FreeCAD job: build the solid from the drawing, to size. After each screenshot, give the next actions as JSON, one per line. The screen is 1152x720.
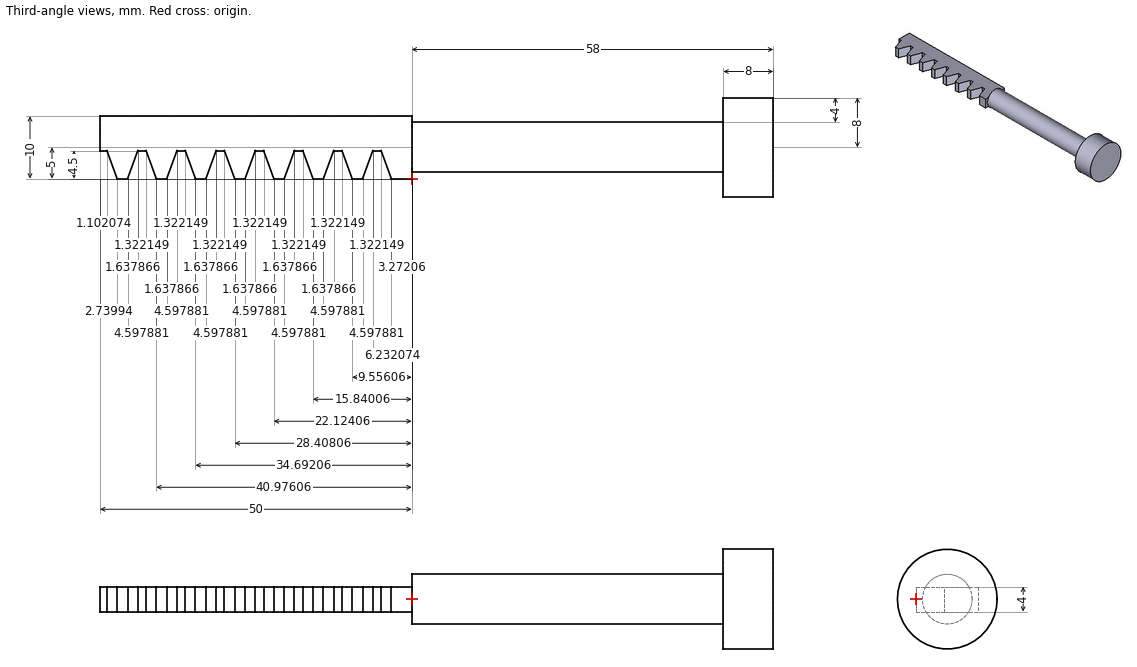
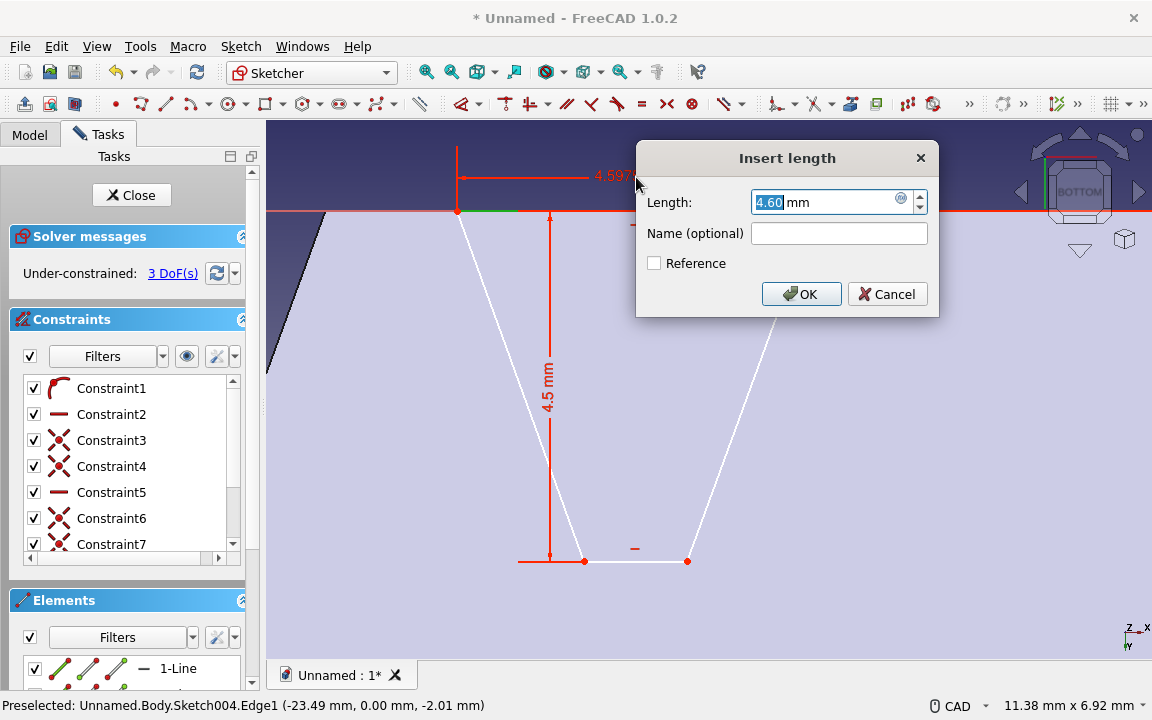
{"action": "type", "text": "4.597881"}
{"action": "key", "text": "Return"}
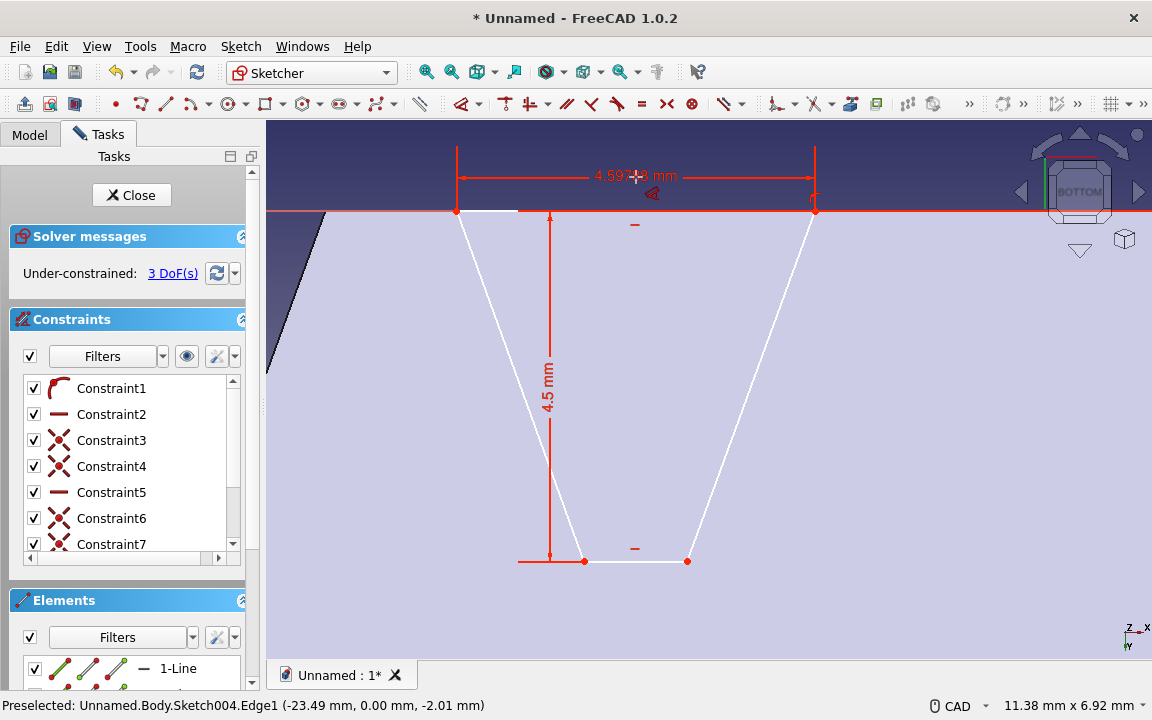
{"action": "left_click", "coordinate": [615, 562]}
{"action": "left_click", "coordinate": [635, 596]}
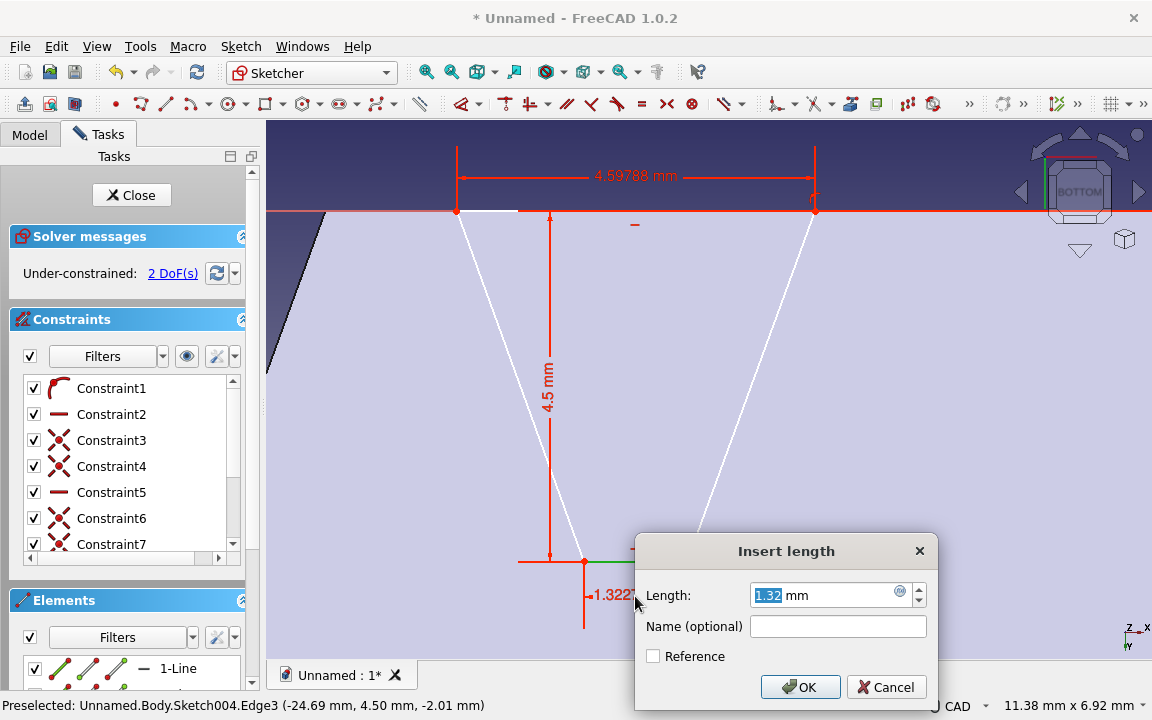
{"action": "type", "text": "1.322149"}
{"action": "key", "text": "Return"}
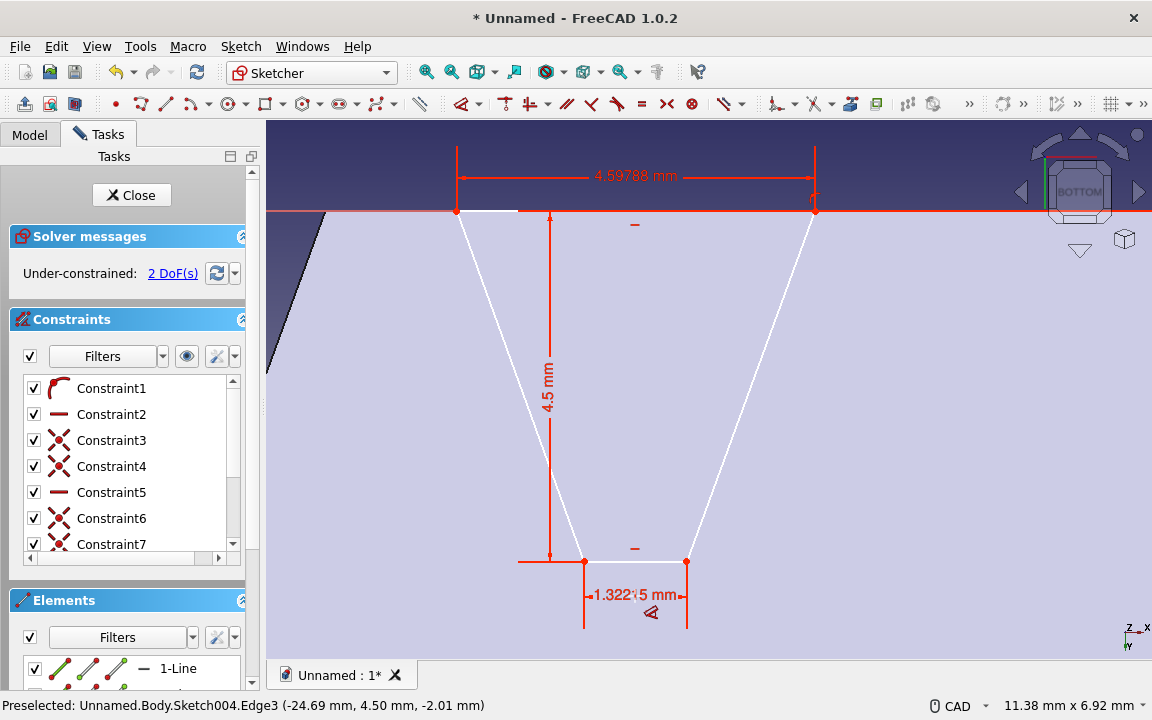
{"action": "left_click", "coordinate": [815, 211]}
{"action": "left_click", "coordinate": [901, 177]}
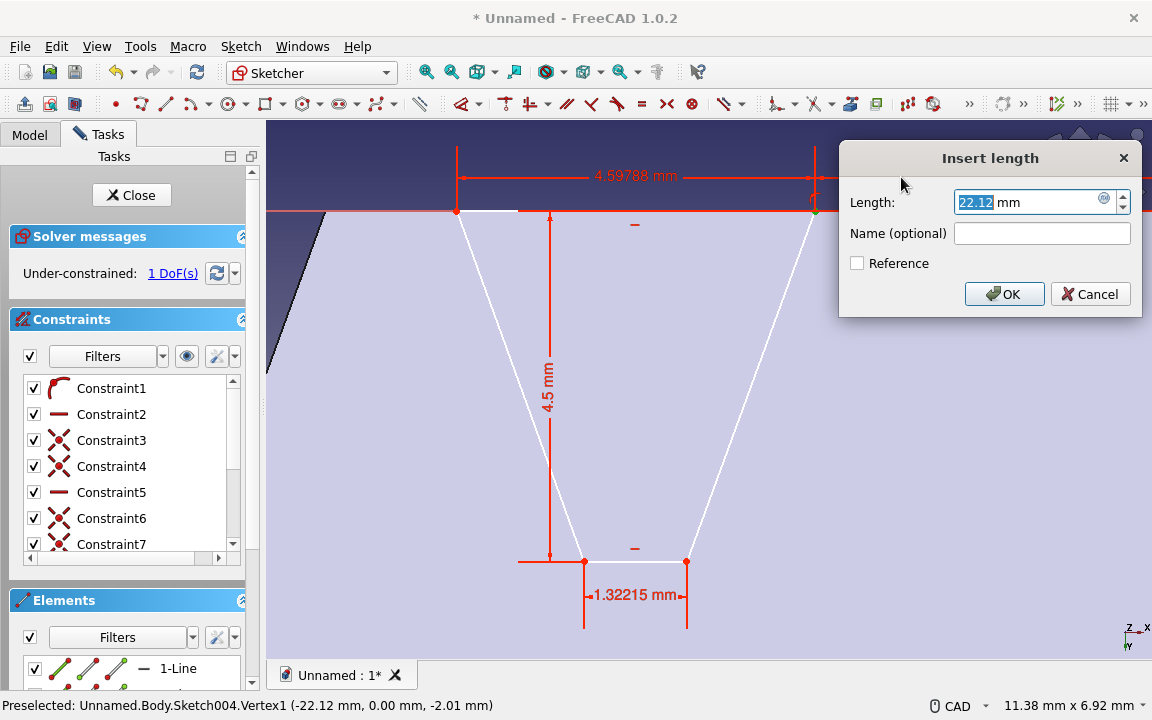
{"action": "type", "text": "22.12406"}
{"action": "key", "text": "Return"}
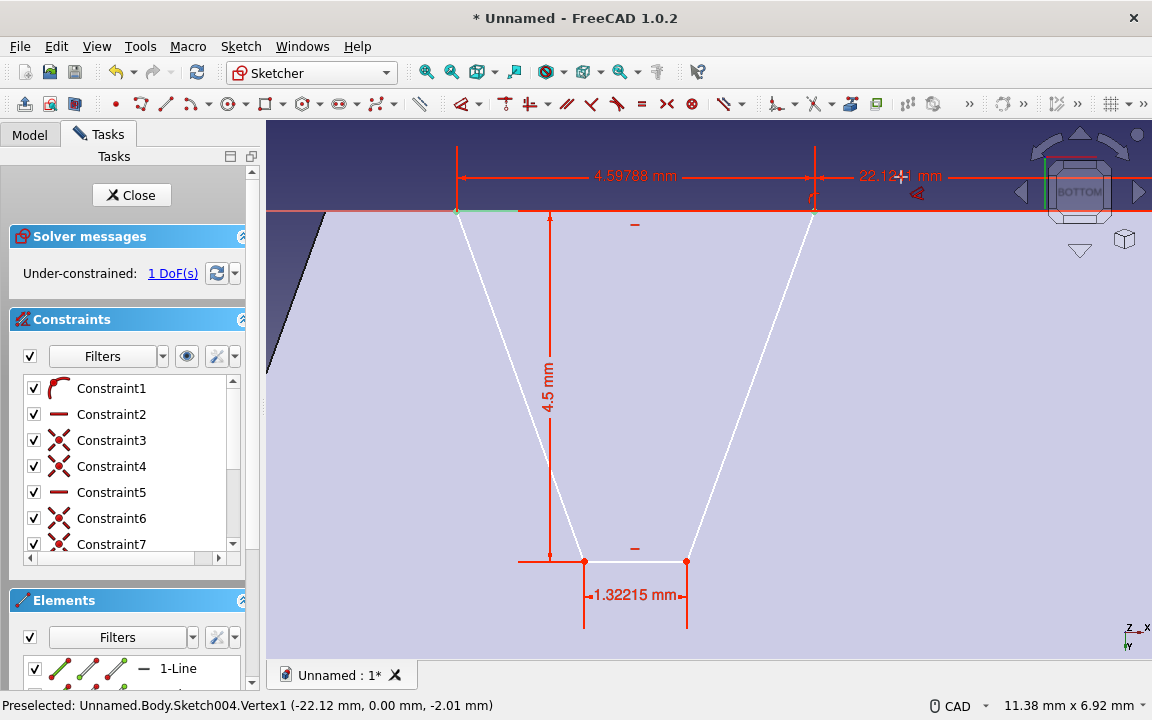
{"action": "left_click", "coordinate": [495, 317]}
{"action": "left_click", "coordinate": [520, 596]}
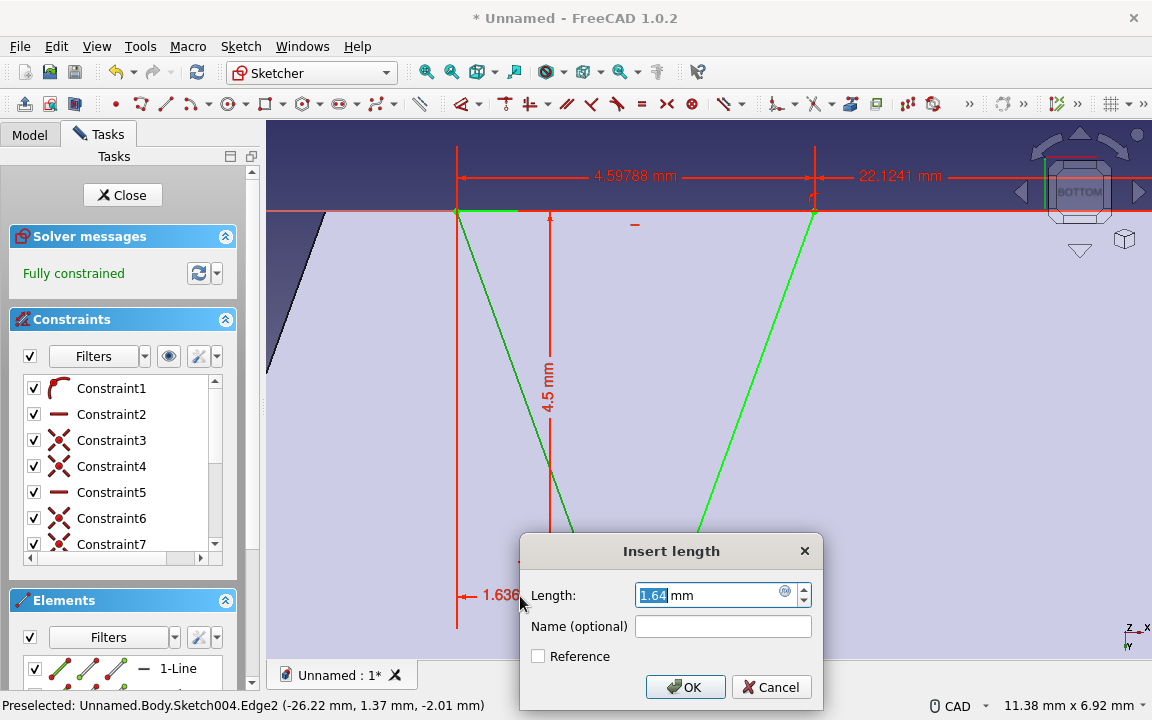
{"action": "type", "text": "1.637866"}
{"action": "key", "text": "Return"}
{"action": "key", "text": "Escape"}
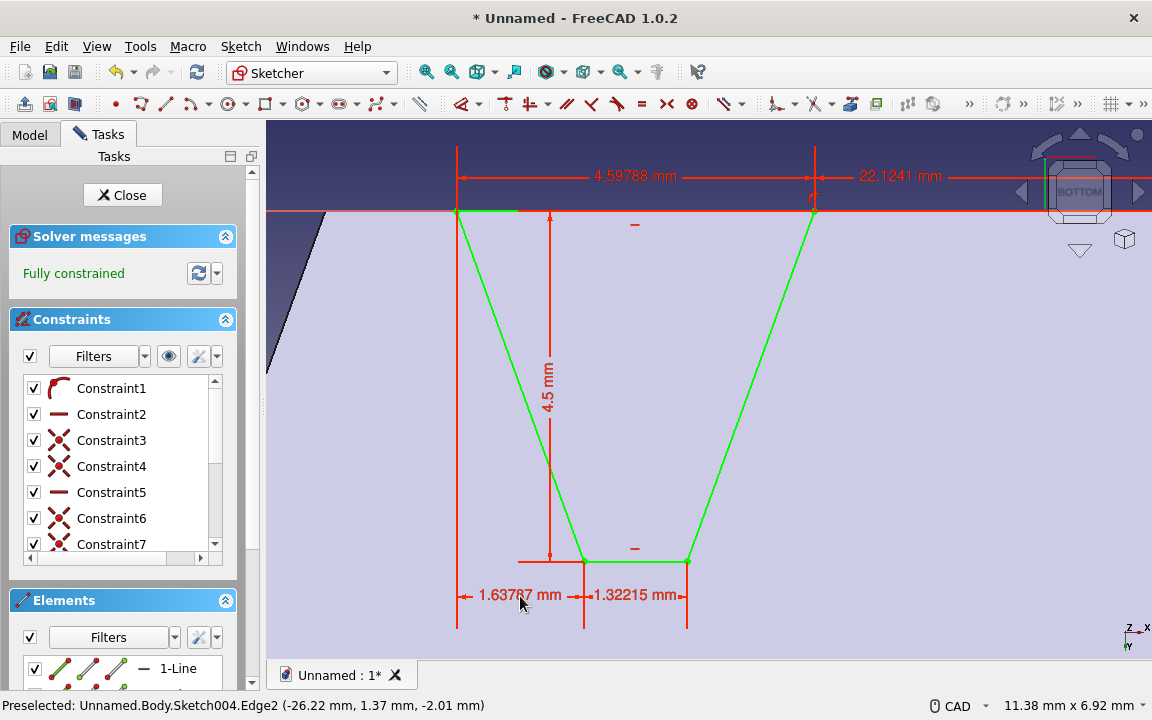
{"action": "left_click", "coordinate": [123, 195]}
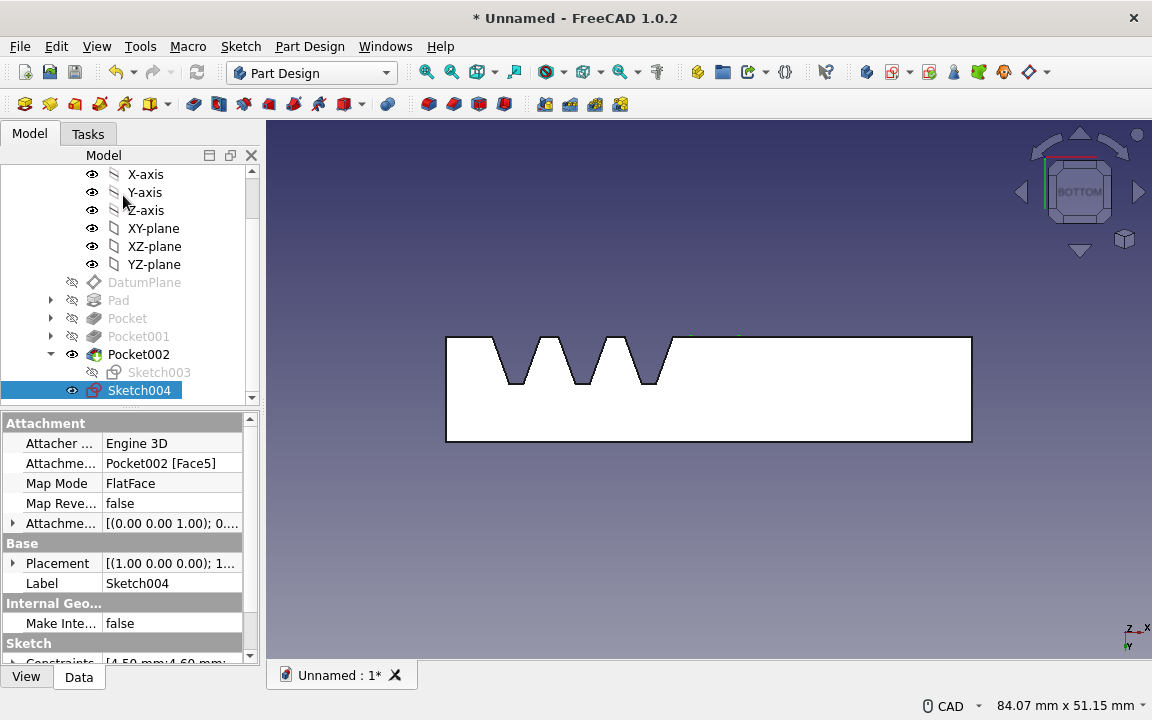
{"action": "left_click", "coordinate": [194, 104]}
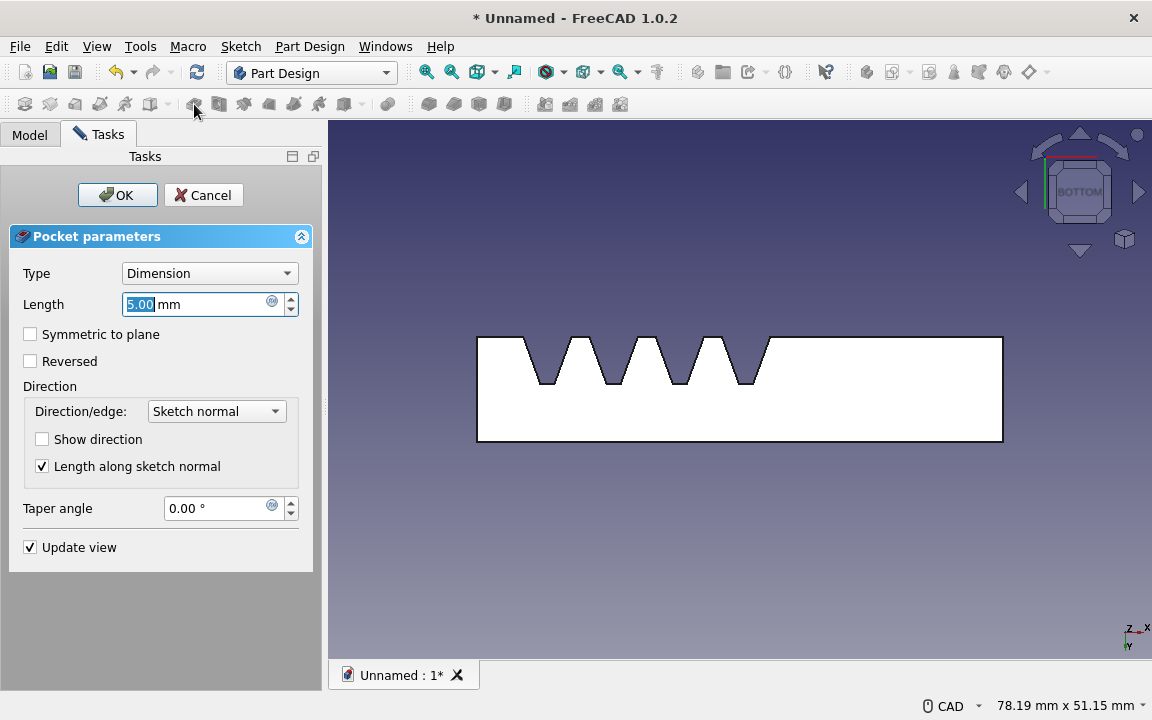
{"action": "left_click", "coordinate": [210, 274]}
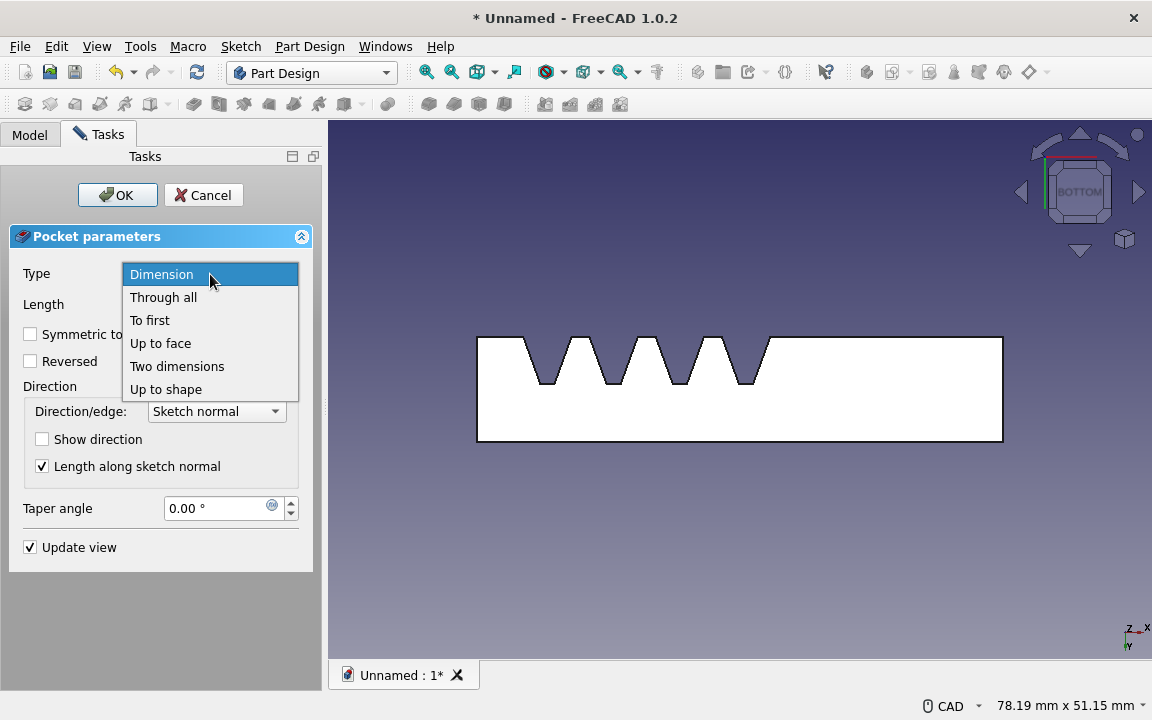
{"action": "left_click", "coordinate": [208, 298]}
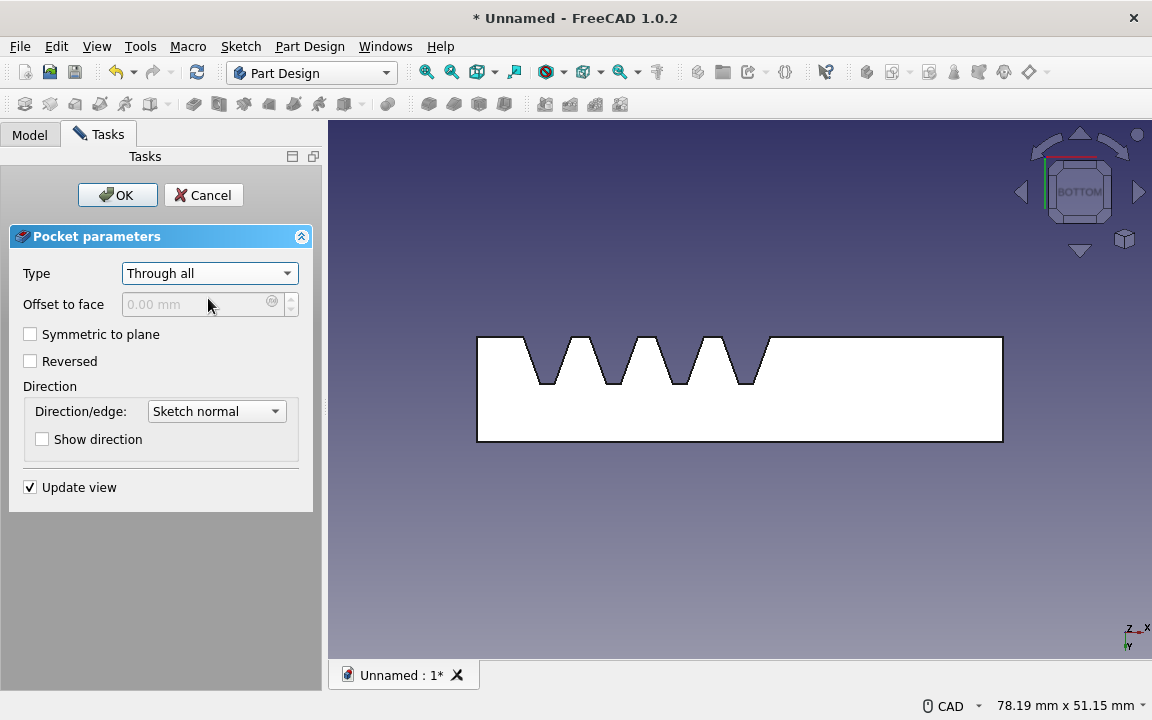
{"action": "left_click", "coordinate": [118, 195]}